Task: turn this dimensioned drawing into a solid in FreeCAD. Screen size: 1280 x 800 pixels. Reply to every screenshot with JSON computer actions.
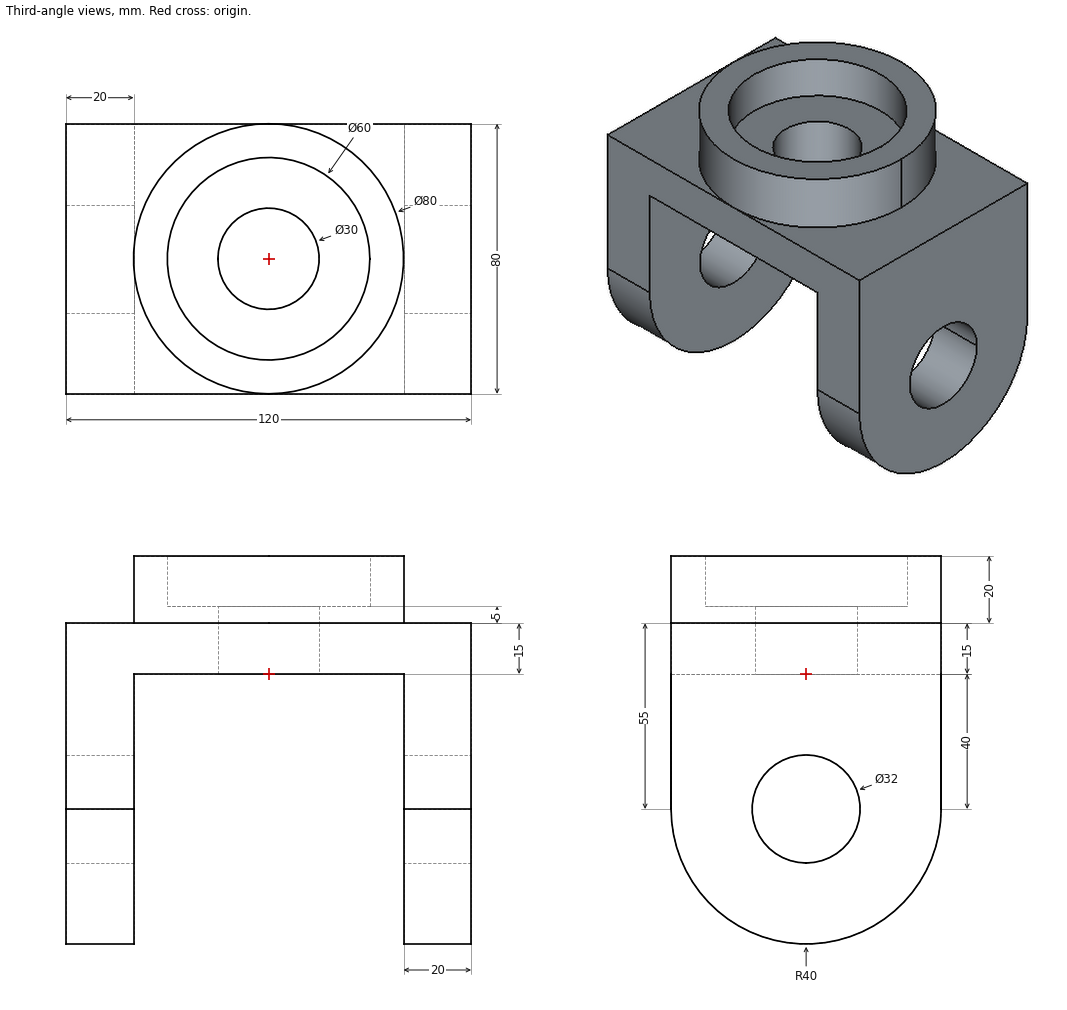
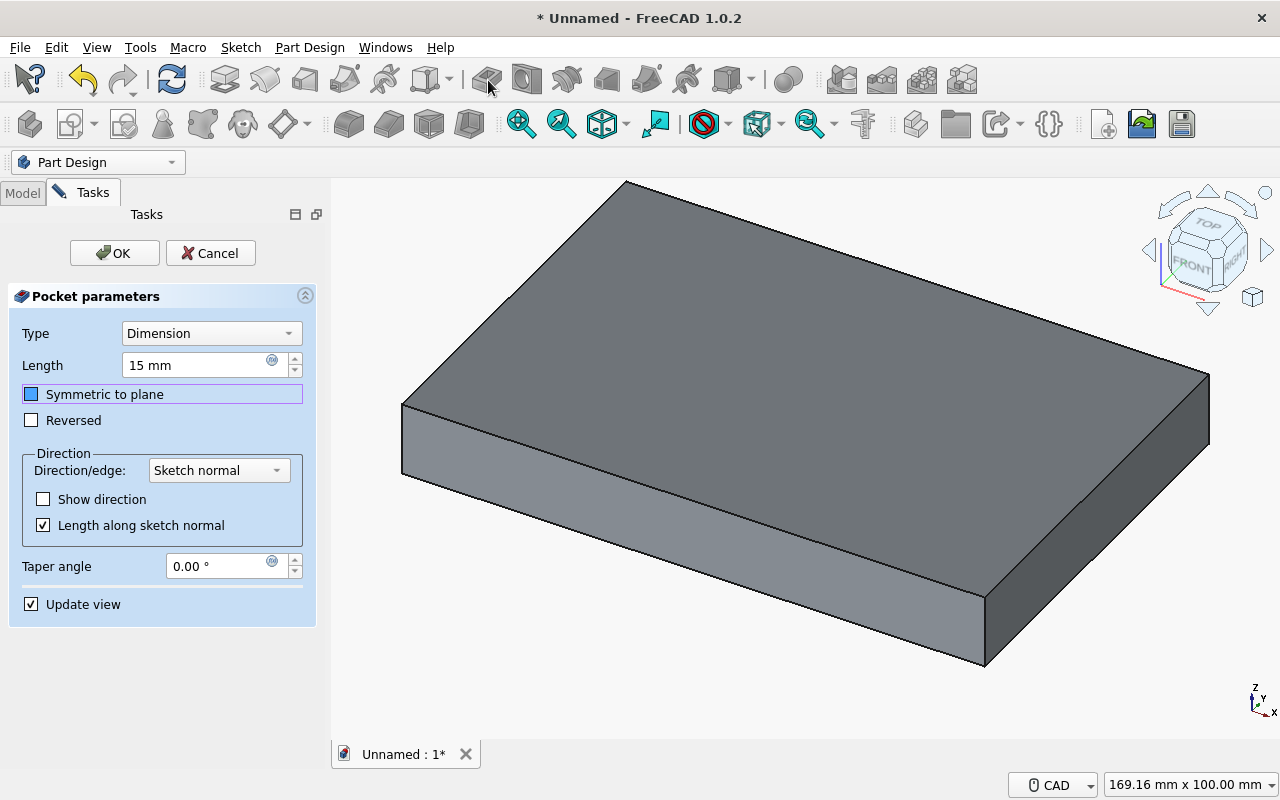
{"action": "left_click", "coordinate": [30, 420]}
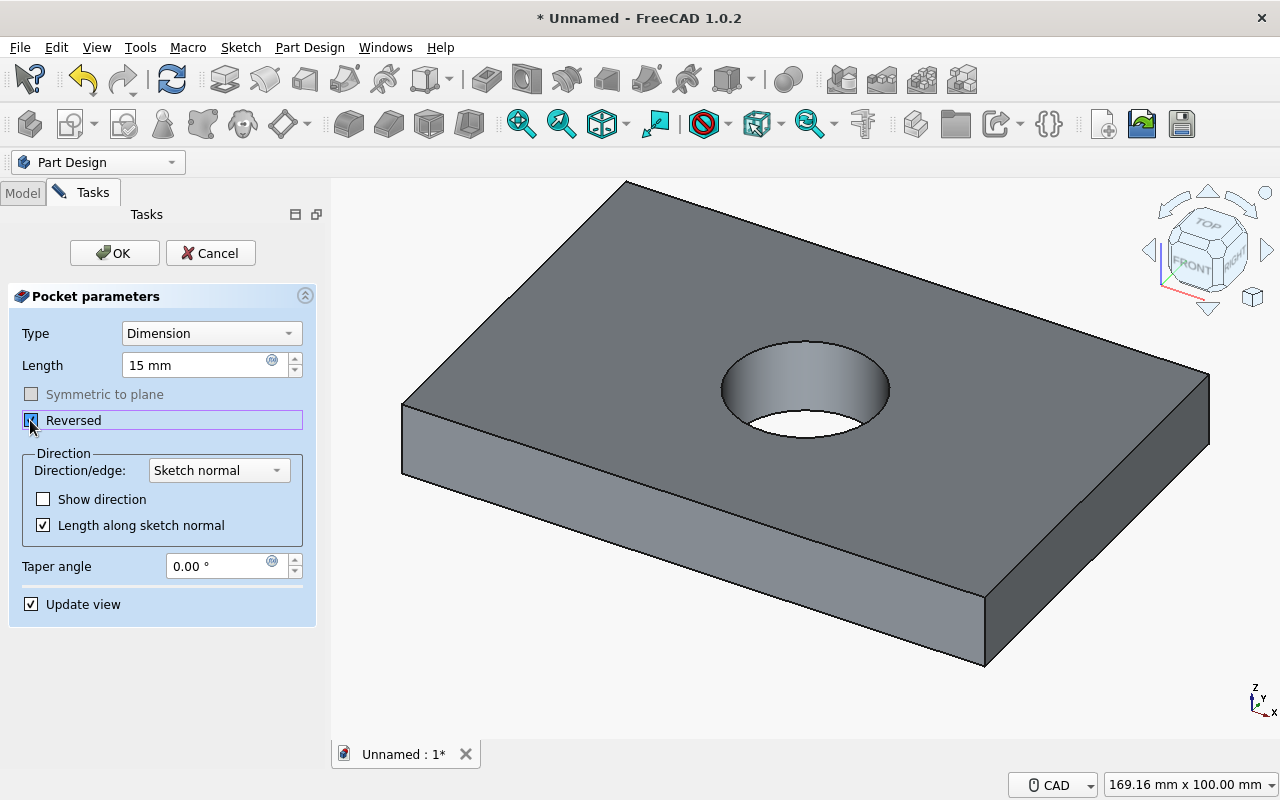
{"action": "left_click", "coordinate": [115, 253]}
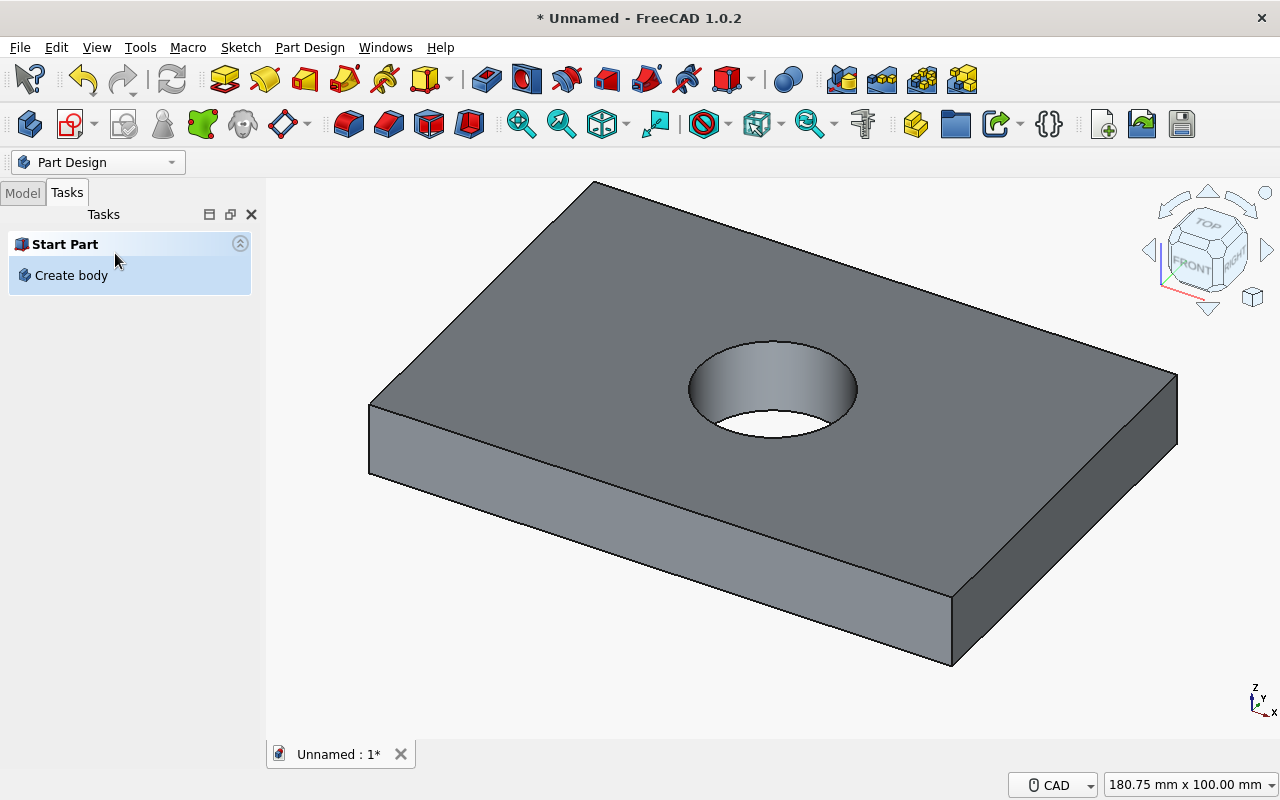
{"action": "left_click", "coordinate": [972, 412]}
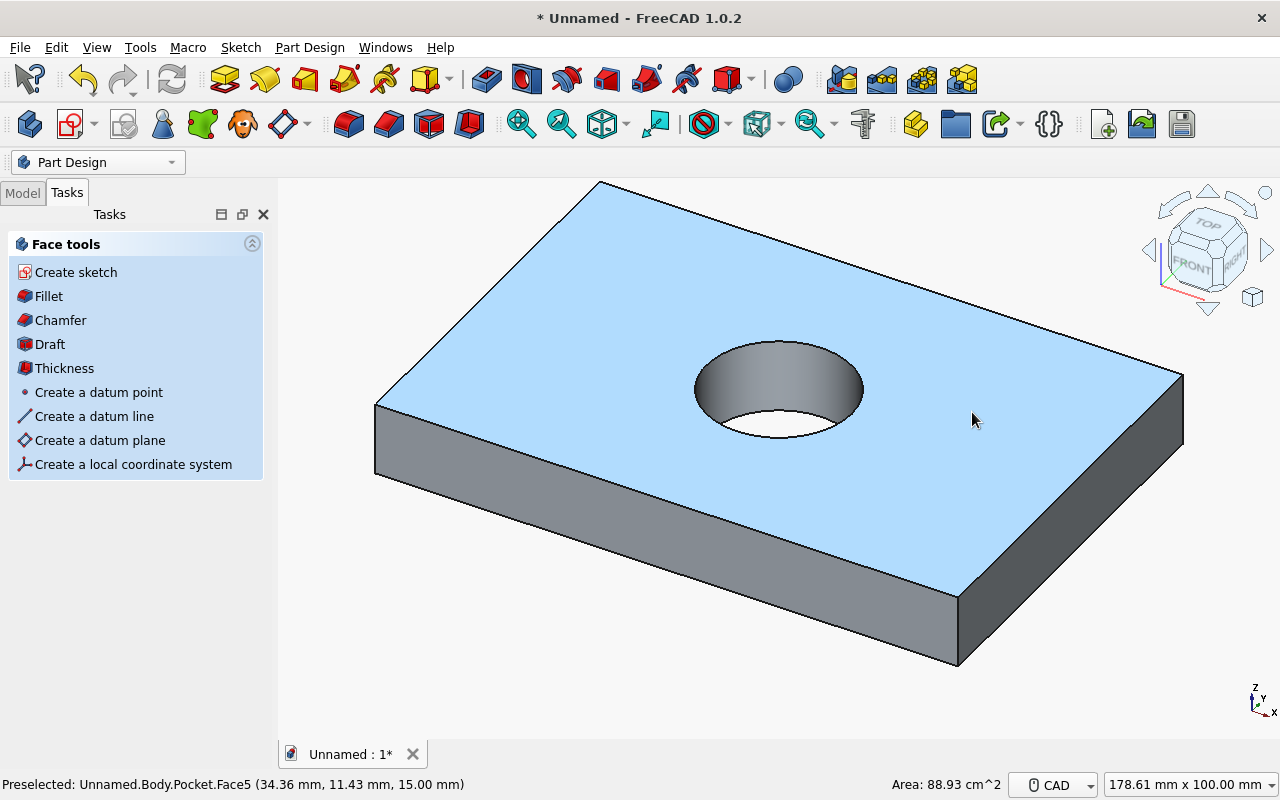
{"action": "left_click", "coordinate": [70, 124]}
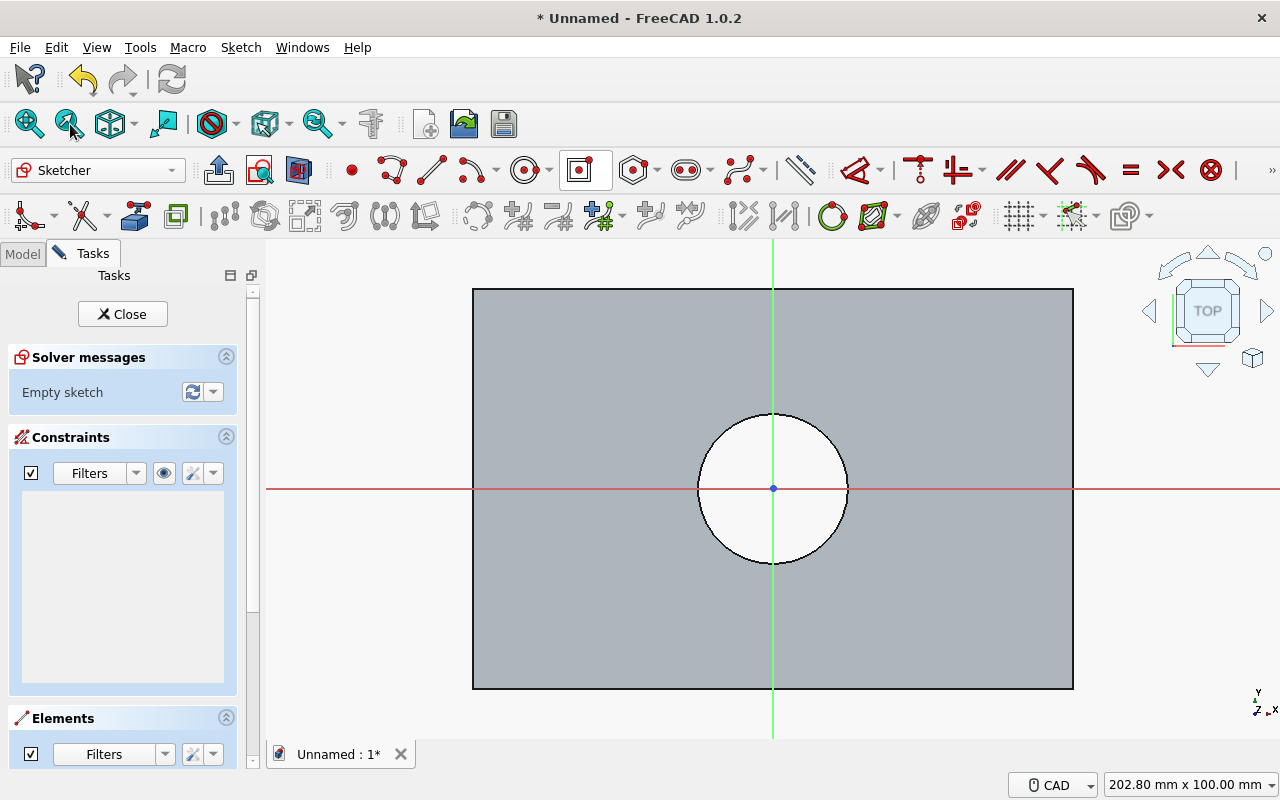
{"action": "scroll", "coordinate": [395, 489], "scroll_direction": "down", "scroll_amount": 1}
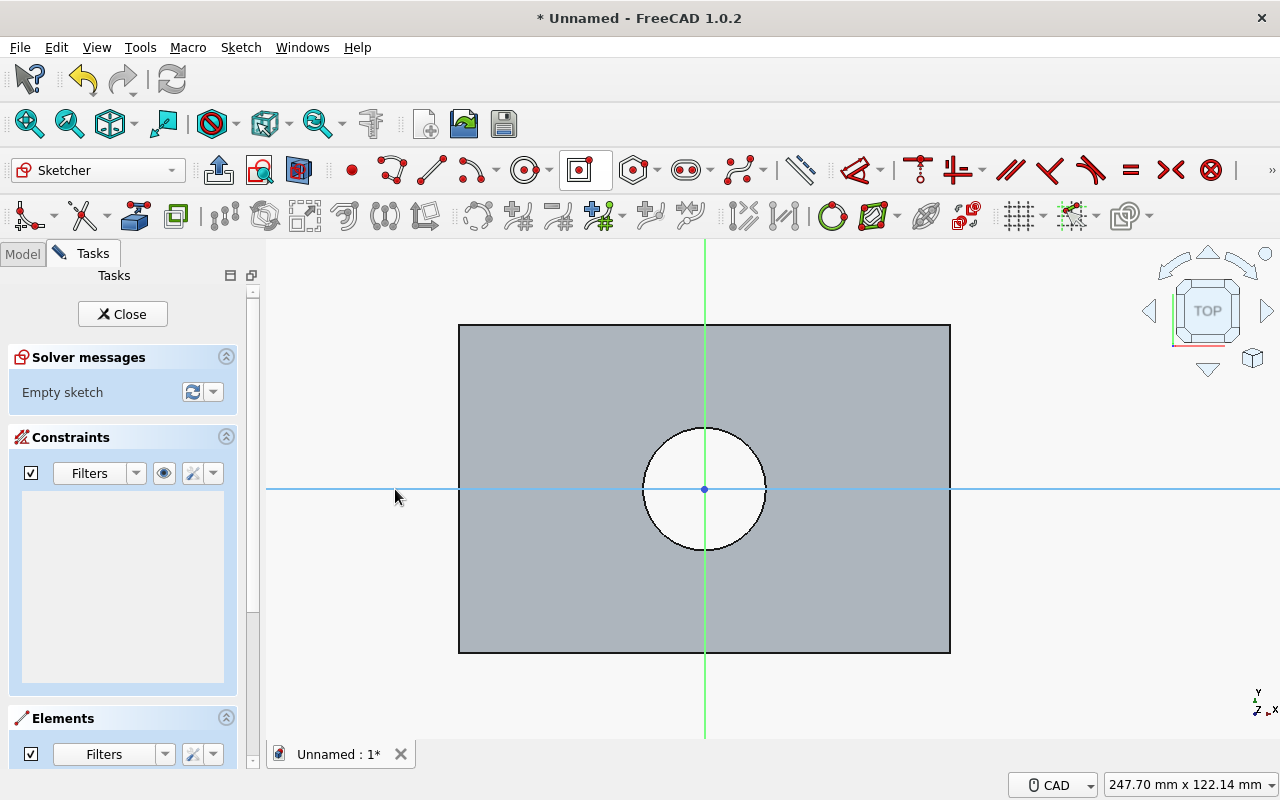
{"action": "key", "text": "g c"}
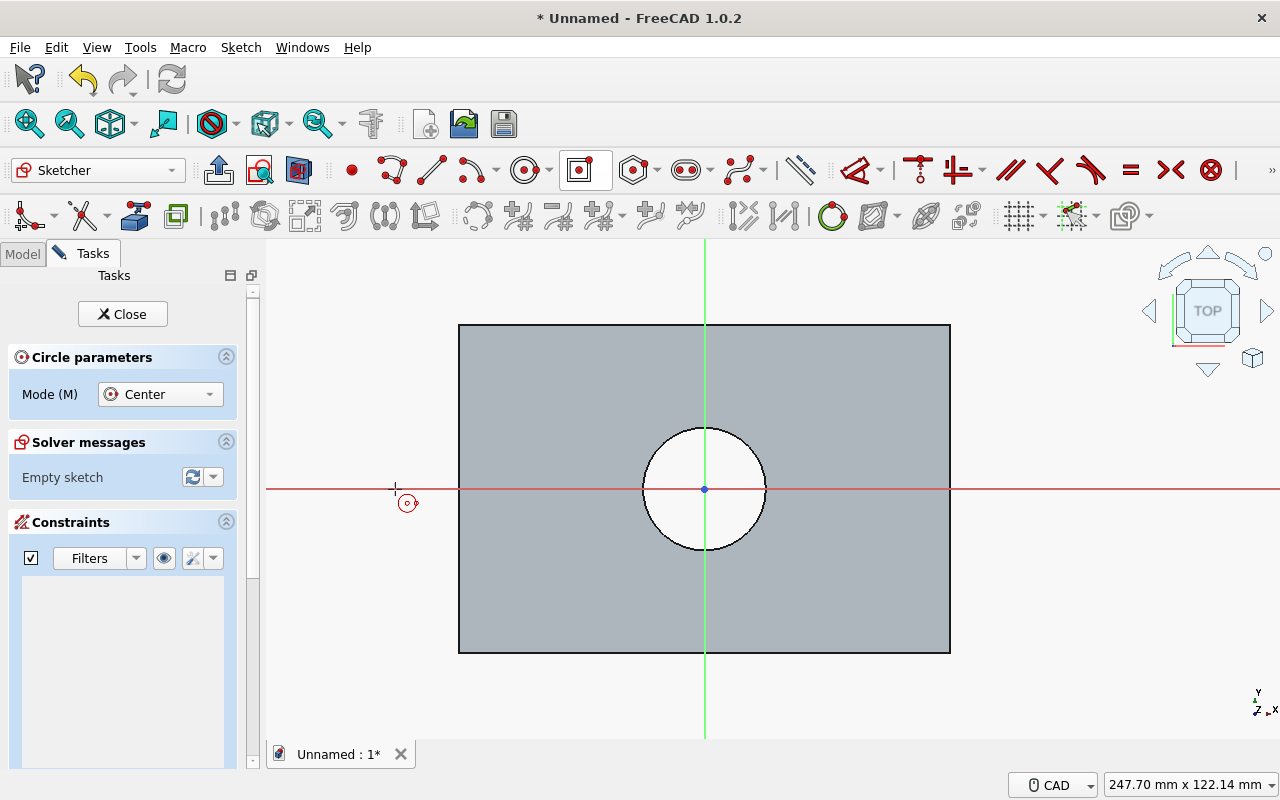
{"action": "left_click", "coordinate": [705, 489]}
{"action": "left_click", "coordinate": [820, 373]}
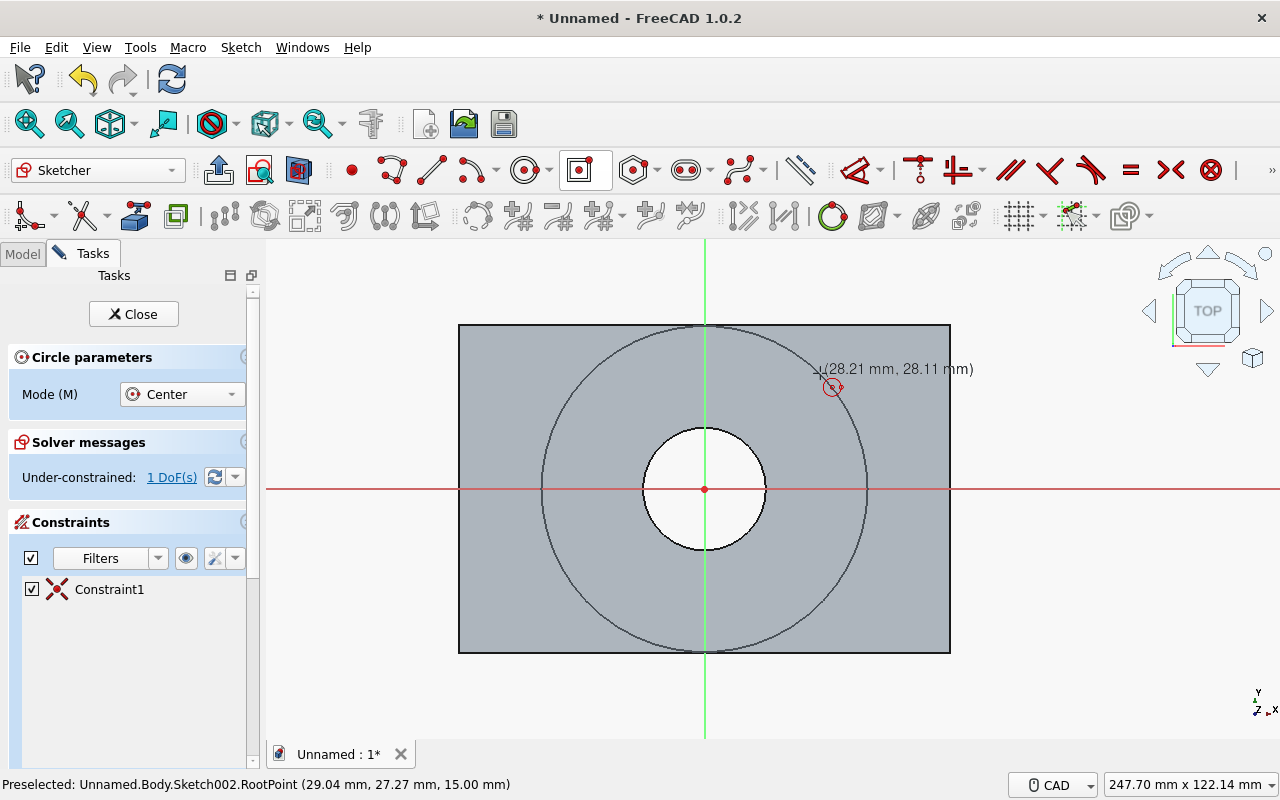
{"action": "left_click", "coordinate": [705, 489]}
{"action": "left_click", "coordinate": [791, 402]}
{"action": "key", "text": "Escape"}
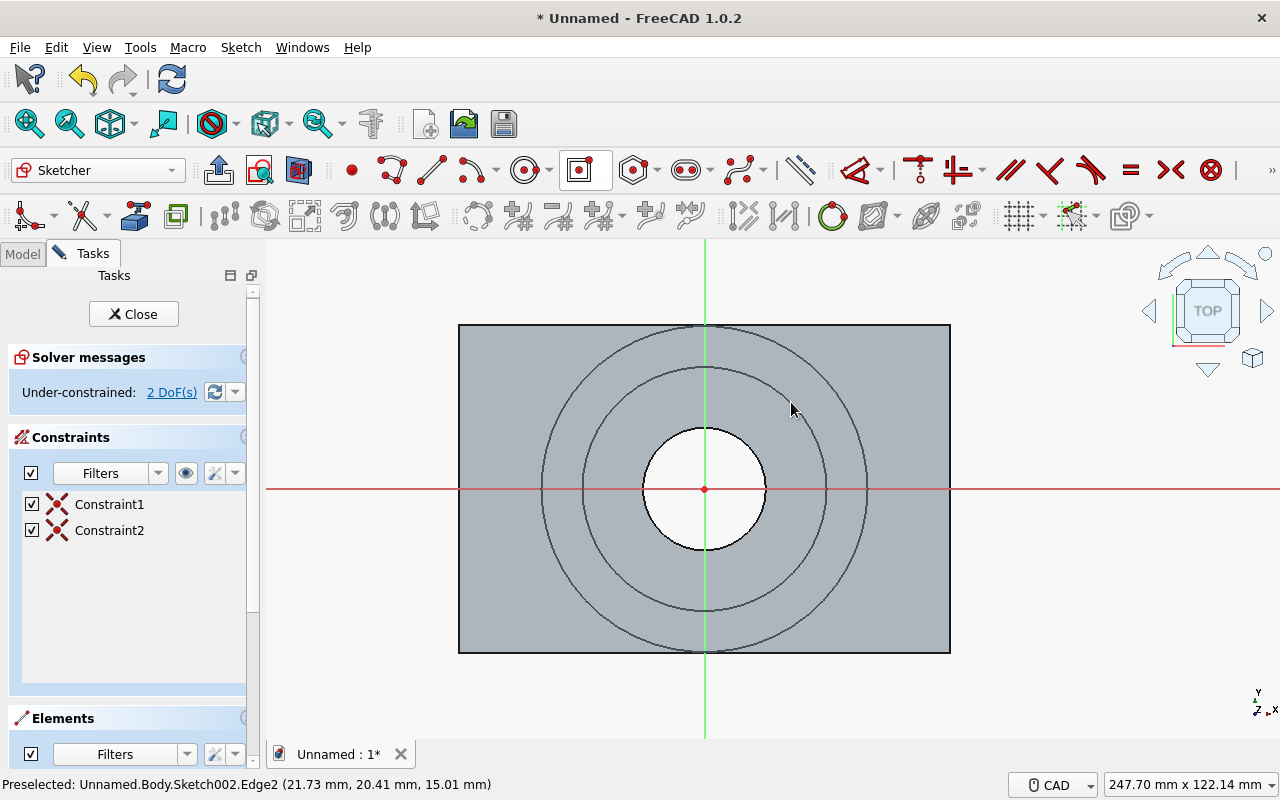
{"action": "left_click", "coordinate": [856, 170]}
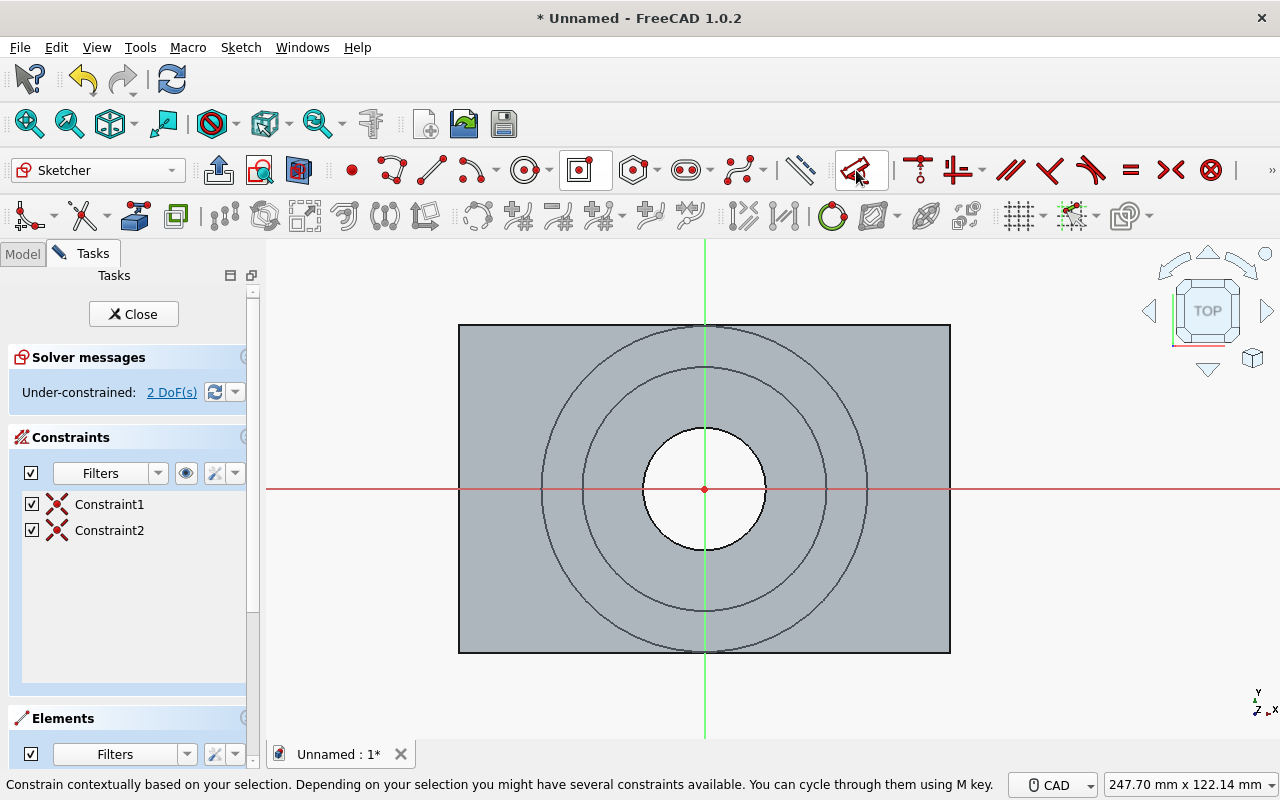
{"action": "left_click", "coordinate": [819, 373]}
{"action": "left_click", "coordinate": [841, 350]}